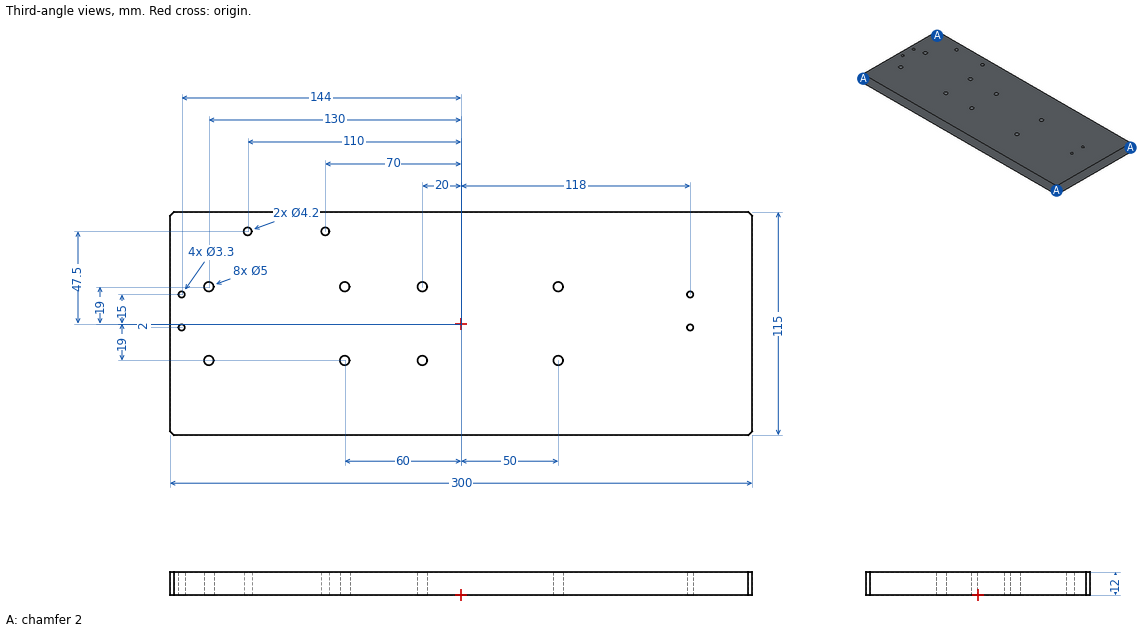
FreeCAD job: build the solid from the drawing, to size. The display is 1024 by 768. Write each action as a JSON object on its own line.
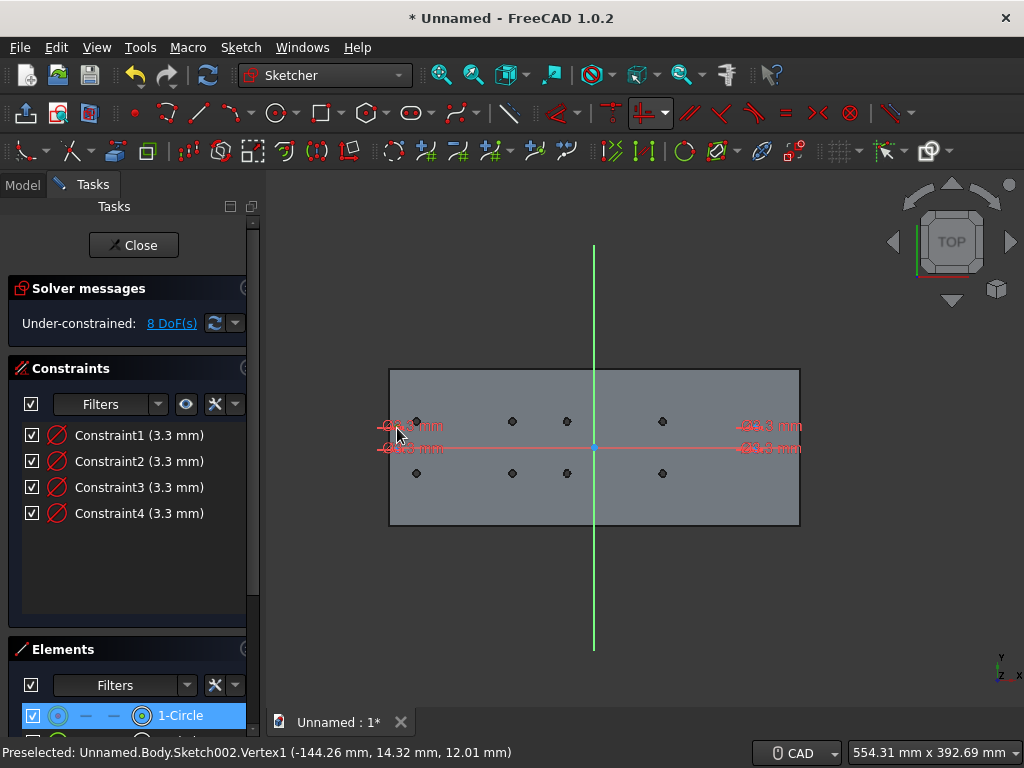
{"action": "left_click", "coordinate": [397, 450]}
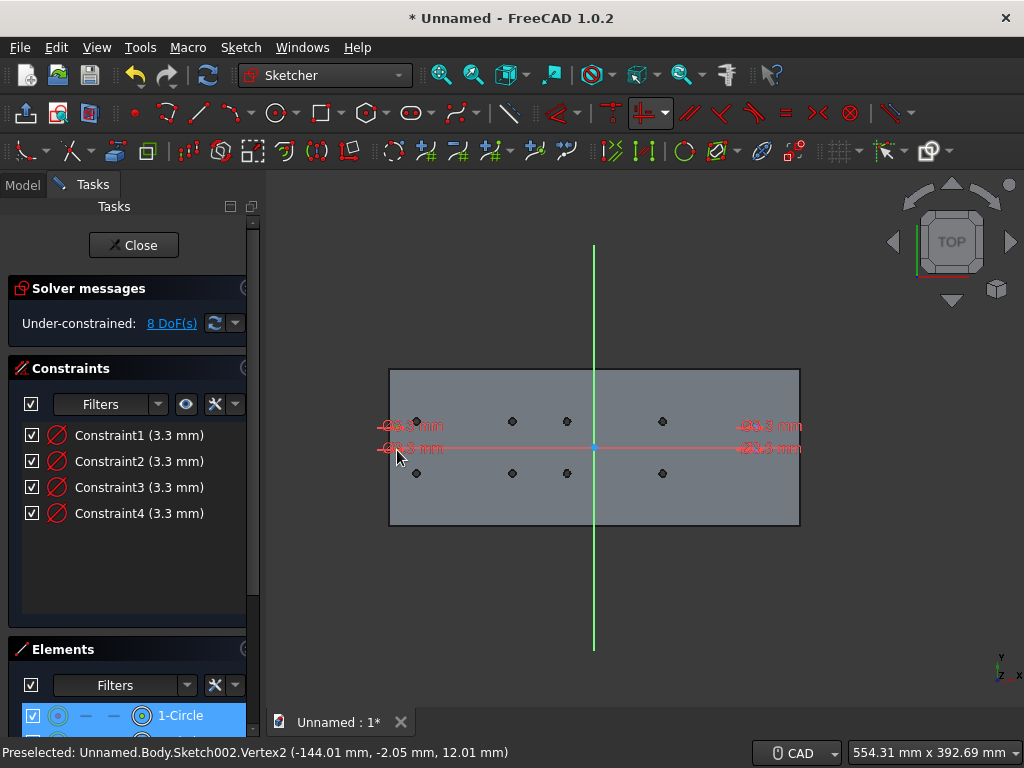
{"action": "key", "text": "v"}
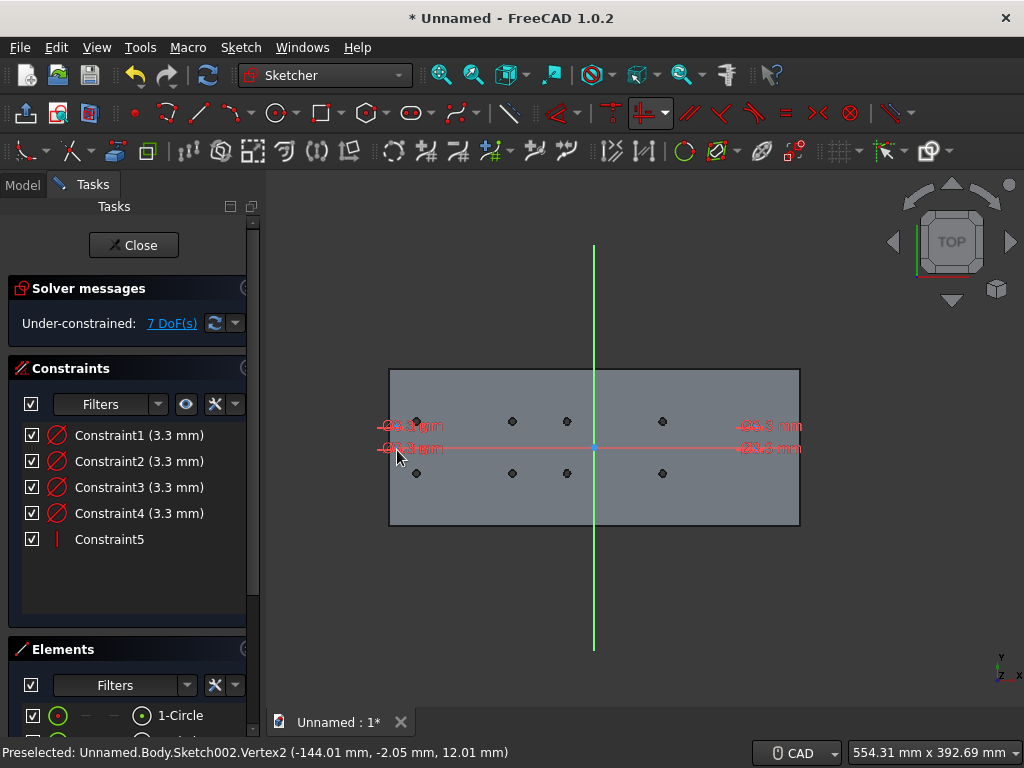
{"action": "left_click", "coordinate": [397, 428]}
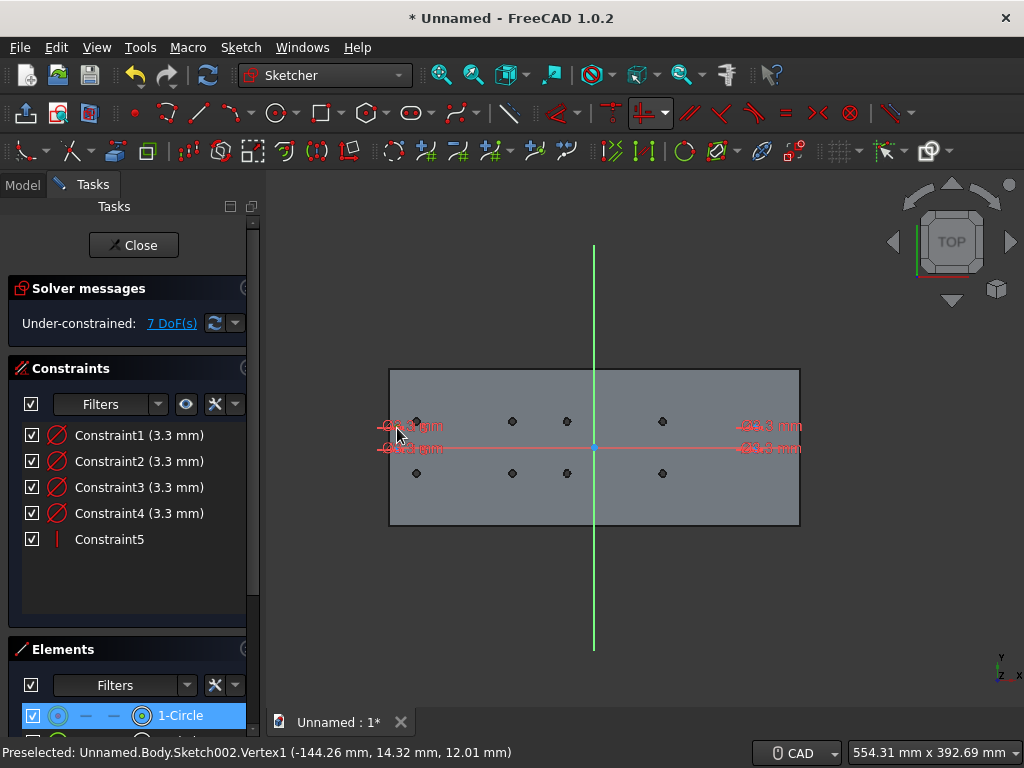
{"action": "left_click", "coordinate": [756, 428]}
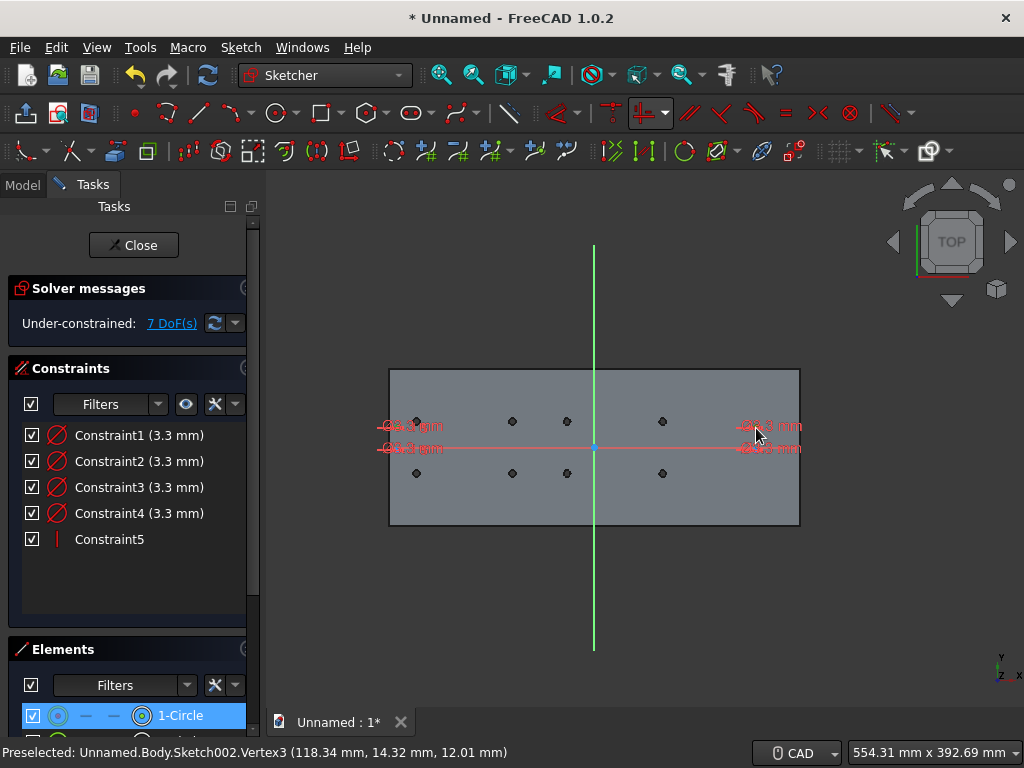
{"action": "left_click", "coordinate": [668, 114]}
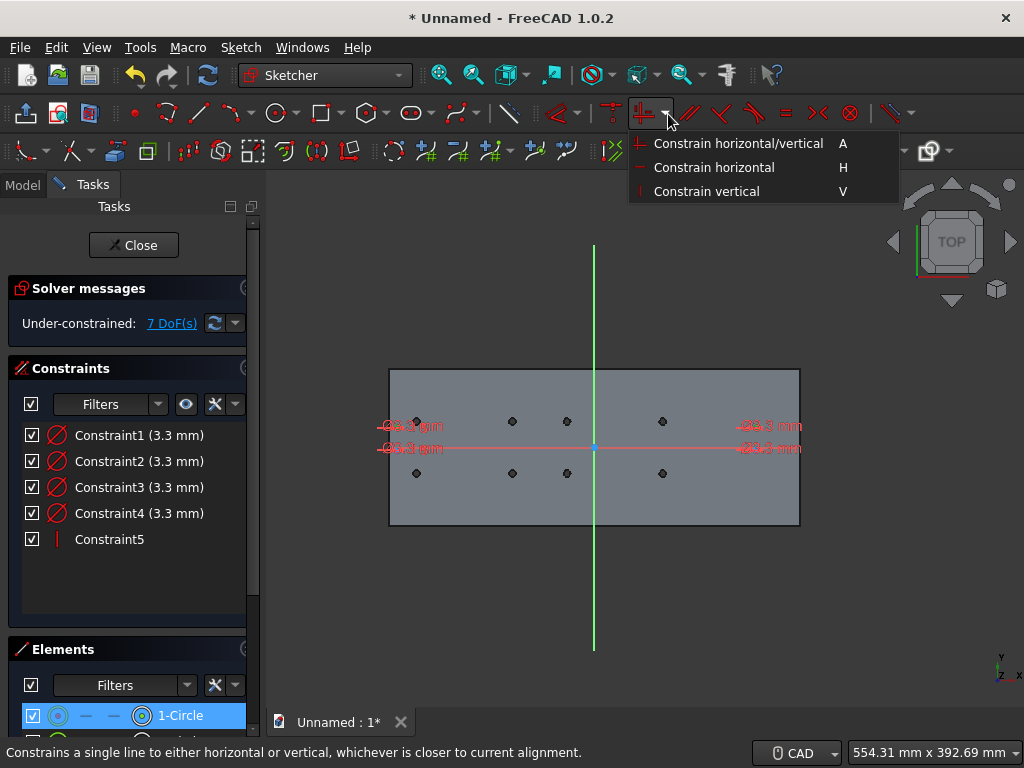
{"action": "left_click", "coordinate": [764, 167]}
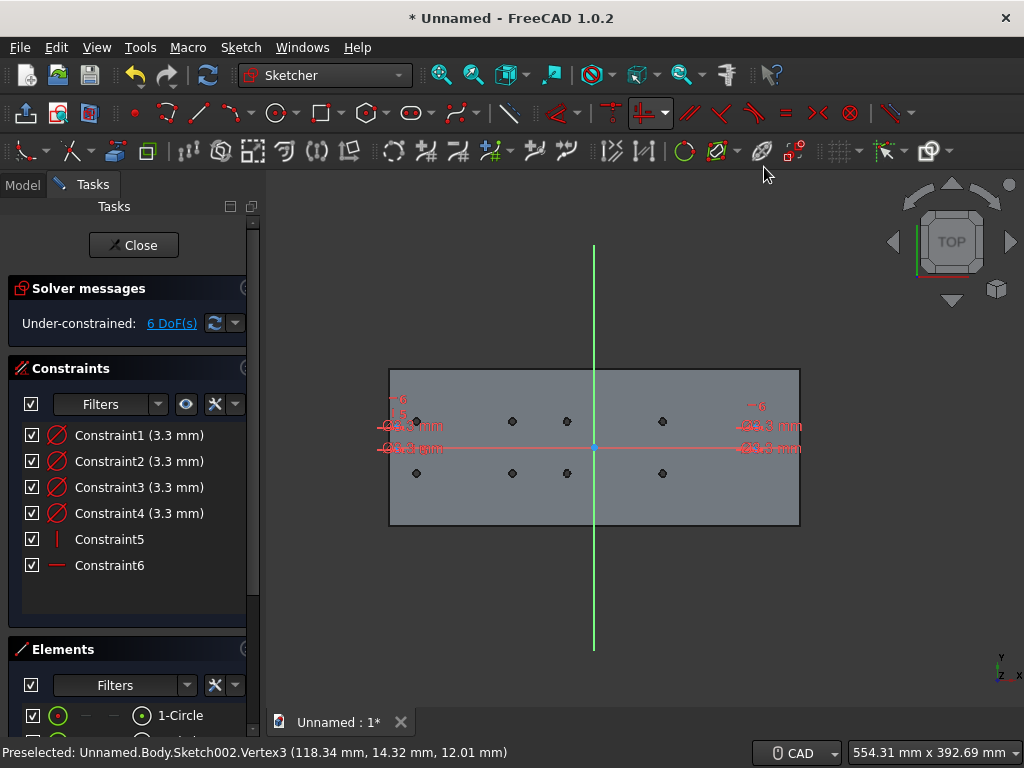
{"action": "left_click", "coordinate": [756, 428]}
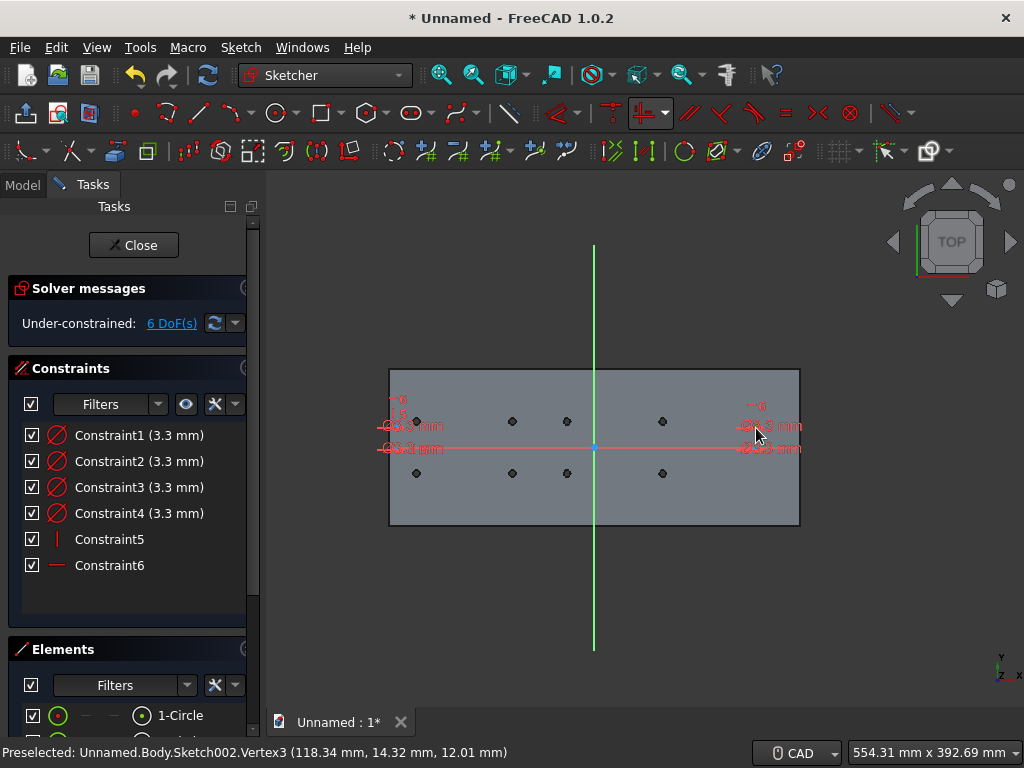
{"action": "left_click", "coordinate": [756, 450]}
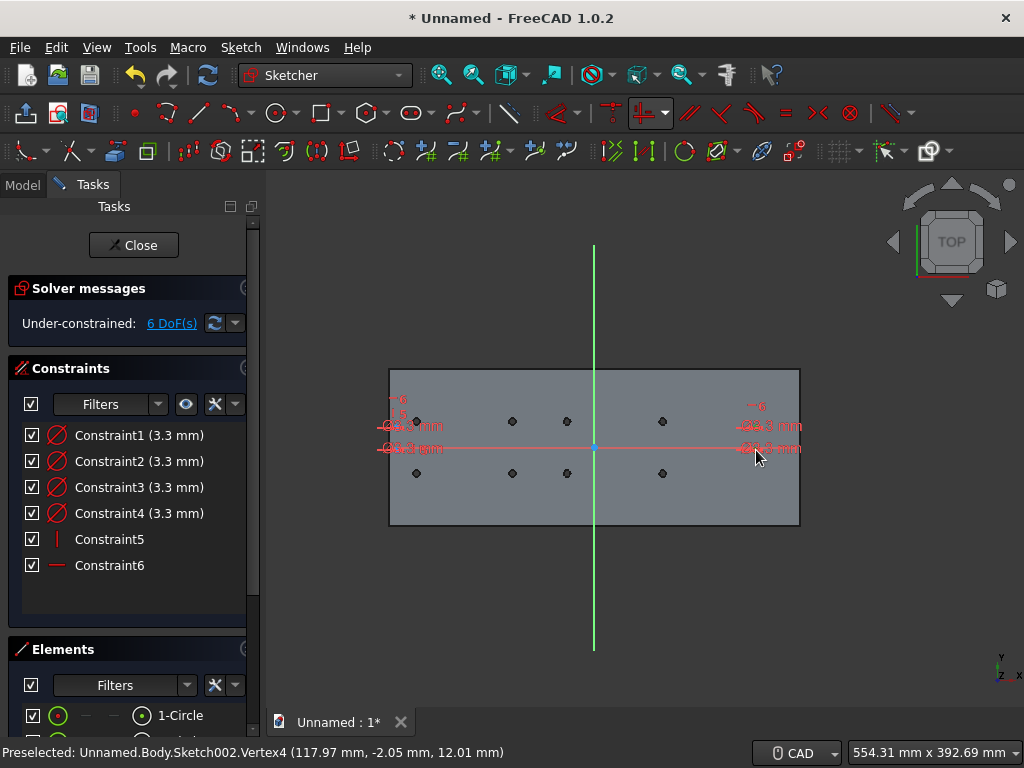
{"action": "left_click", "coordinate": [668, 114]}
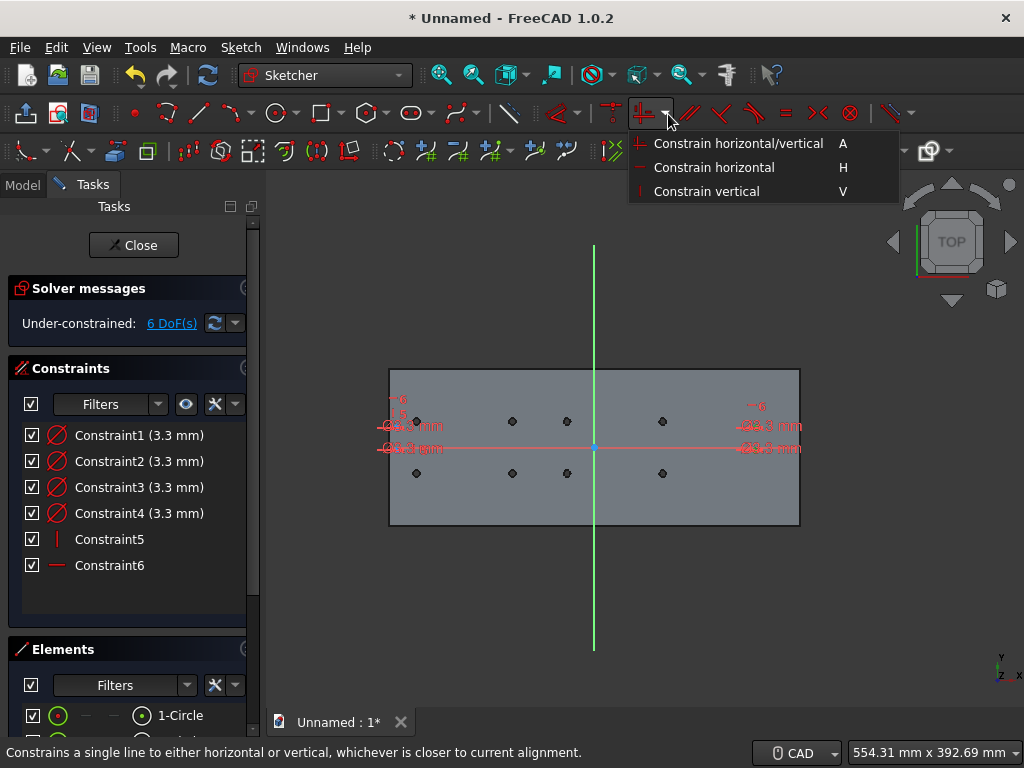
{"action": "left_click", "coordinate": [764, 191]}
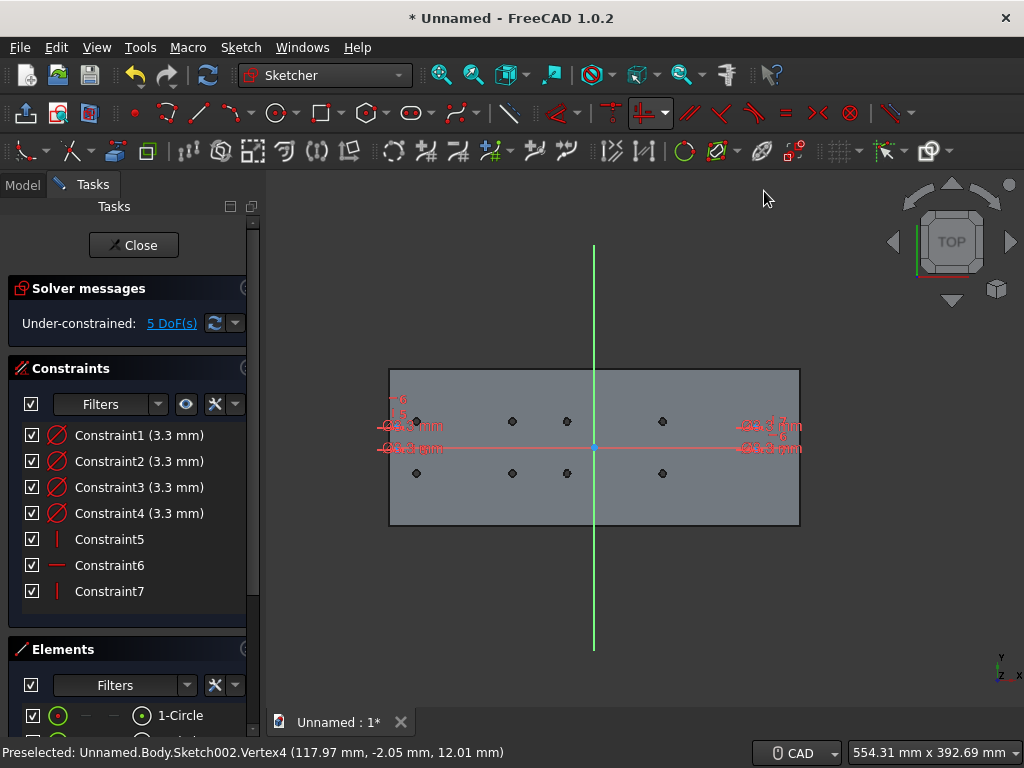
{"action": "left_click", "coordinate": [397, 450]}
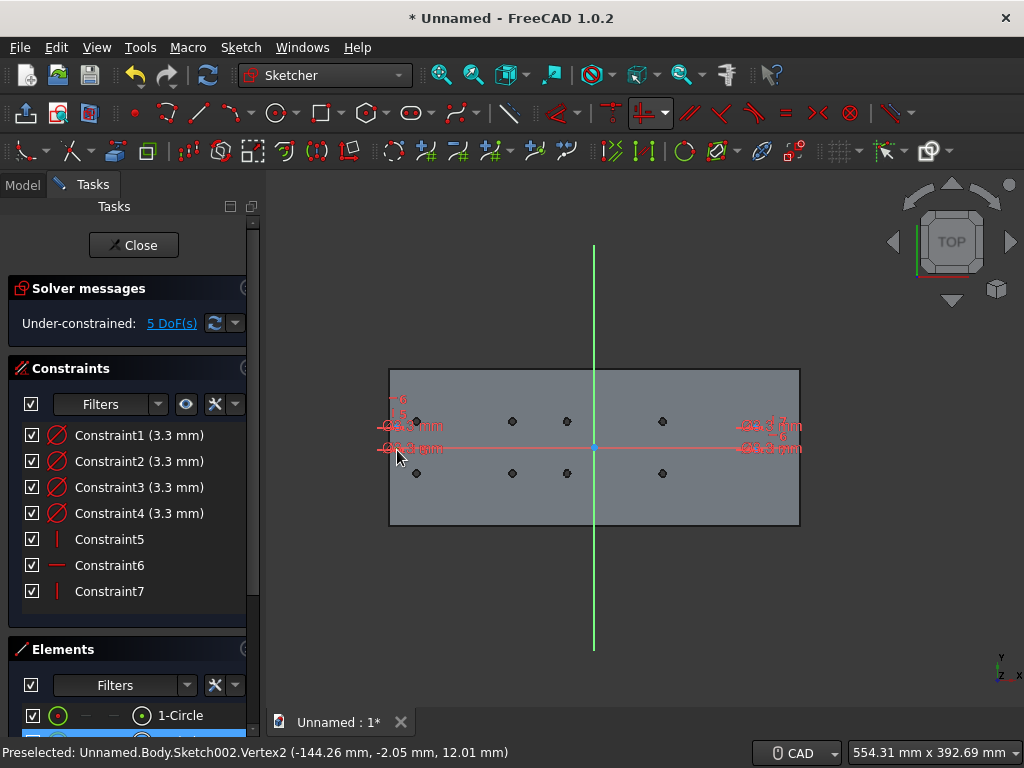
{"action": "left_click", "coordinate": [756, 450]}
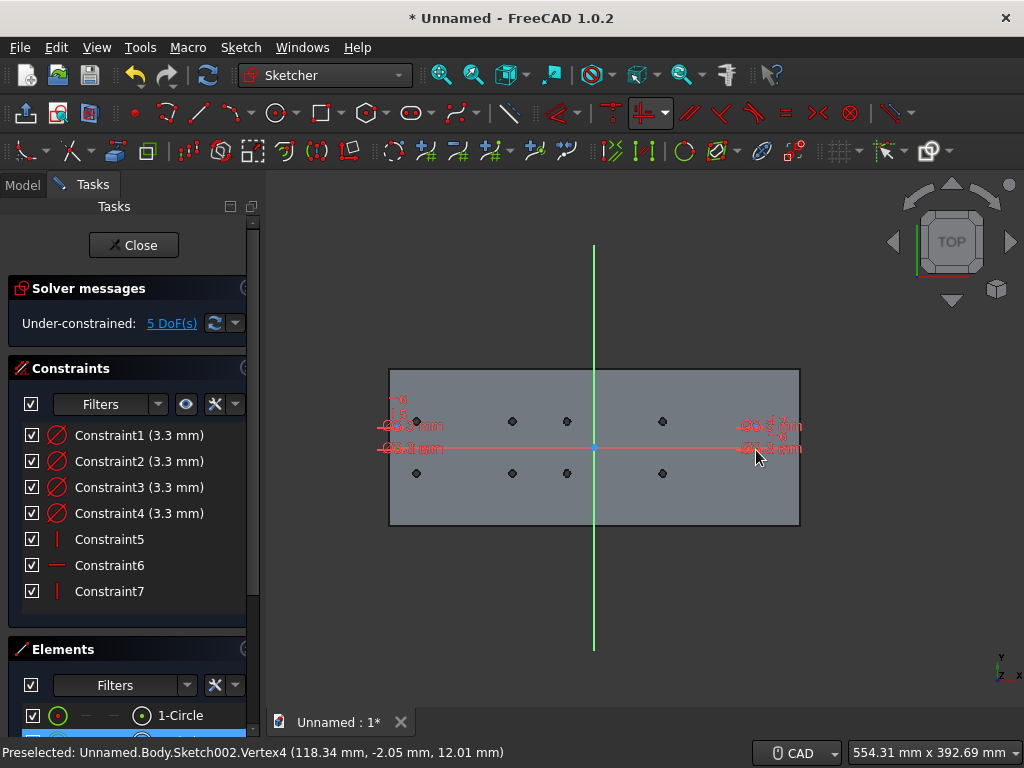
{"action": "left_click", "coordinate": [668, 114]}